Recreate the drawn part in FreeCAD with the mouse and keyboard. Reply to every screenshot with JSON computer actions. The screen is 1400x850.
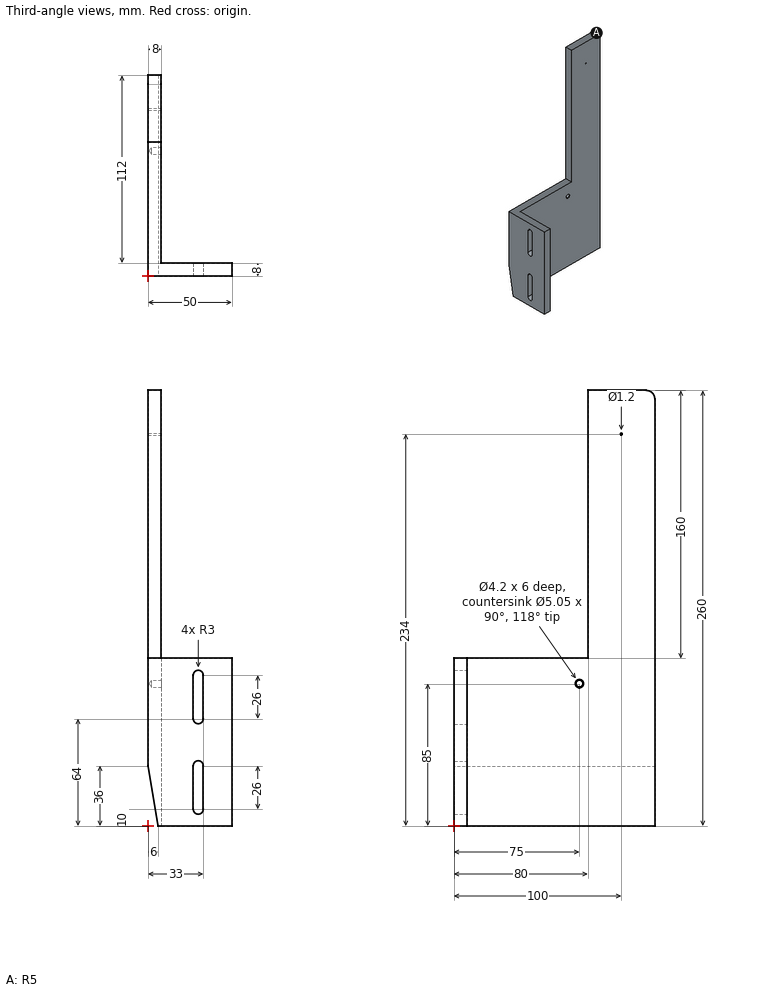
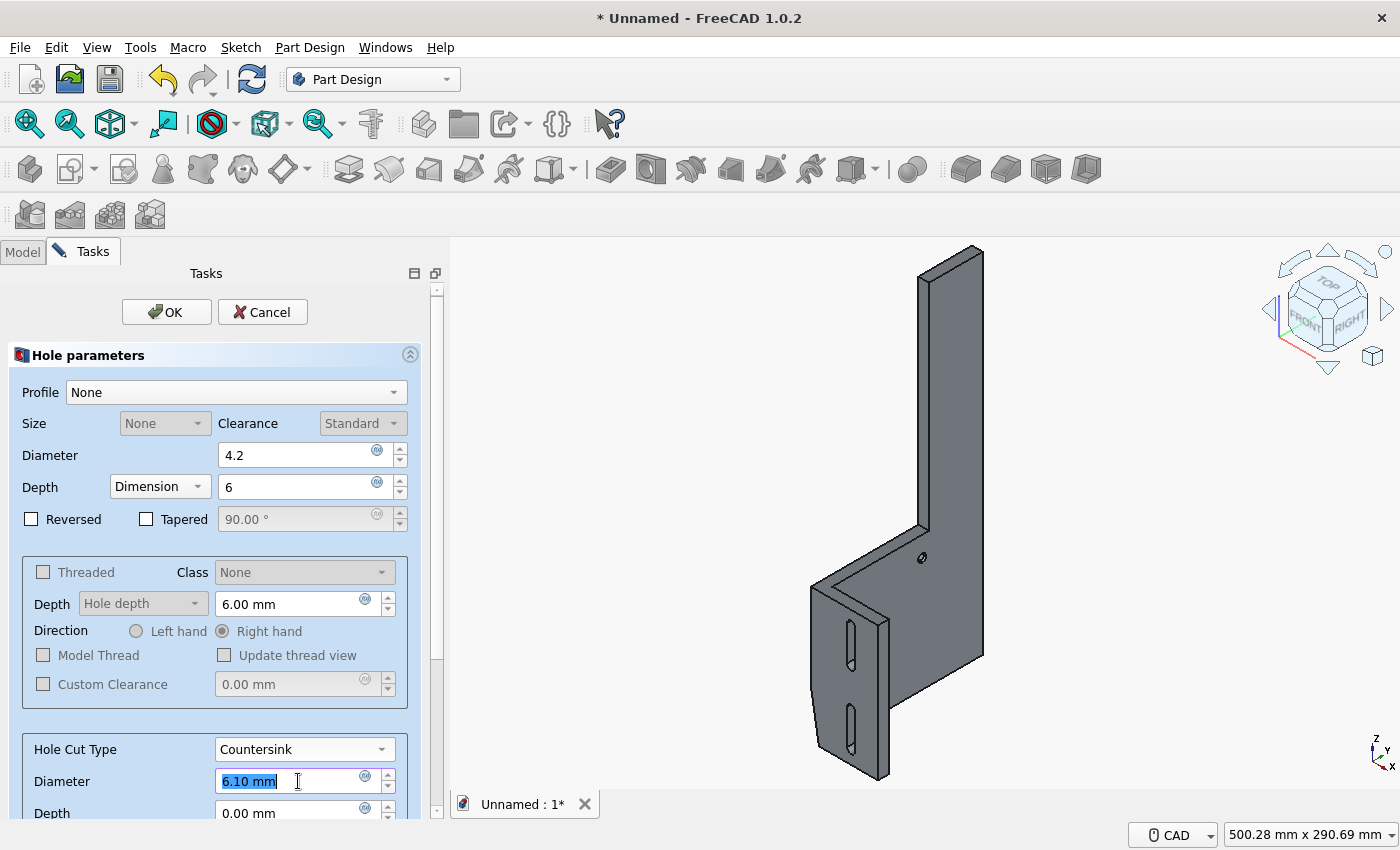
{"action": "type", "text": "5.05"}
{"action": "key", "text": "Tab"}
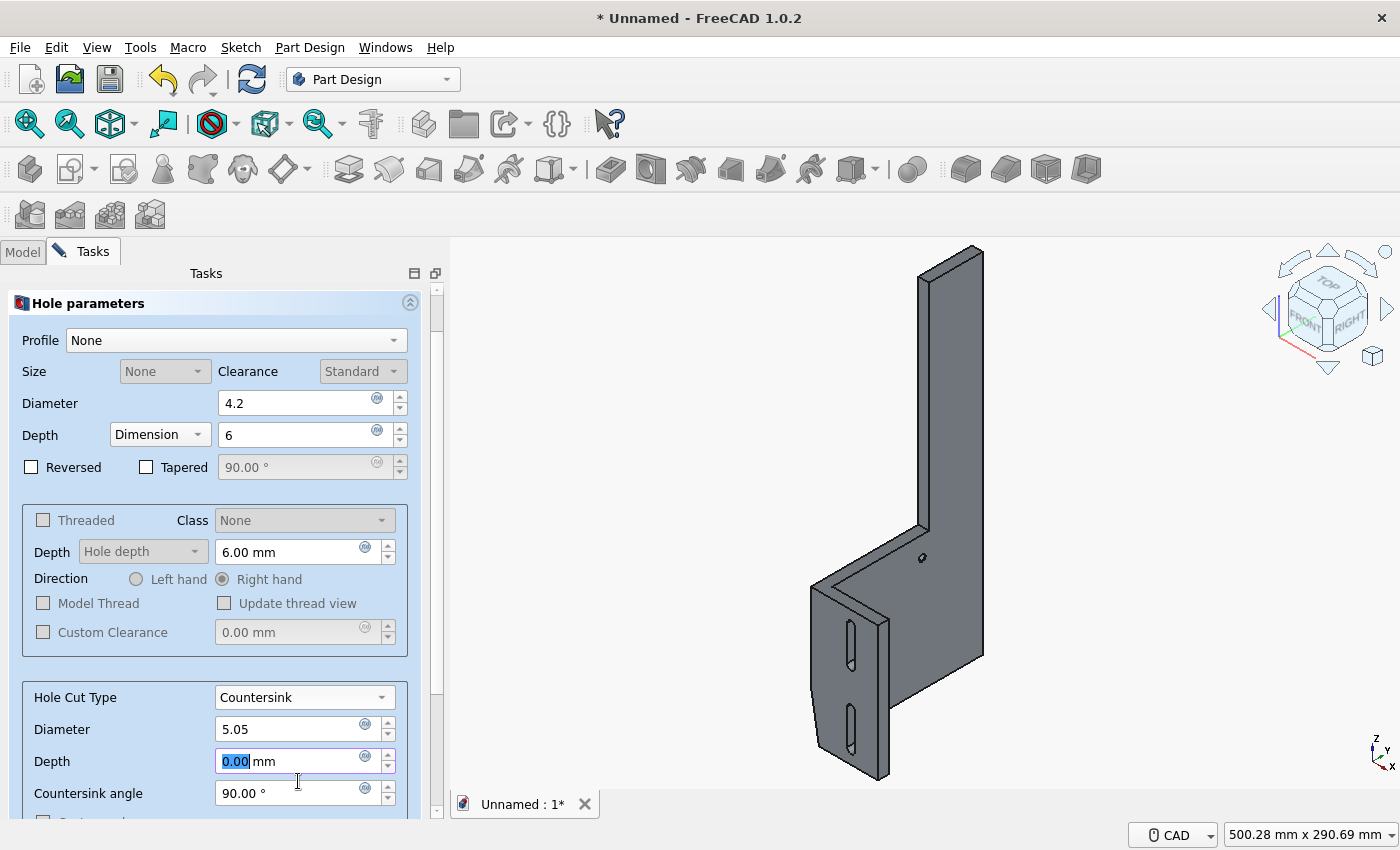
{"action": "scroll", "coordinate": [437, 550], "scroll_direction": "up", "scroll_amount": 2}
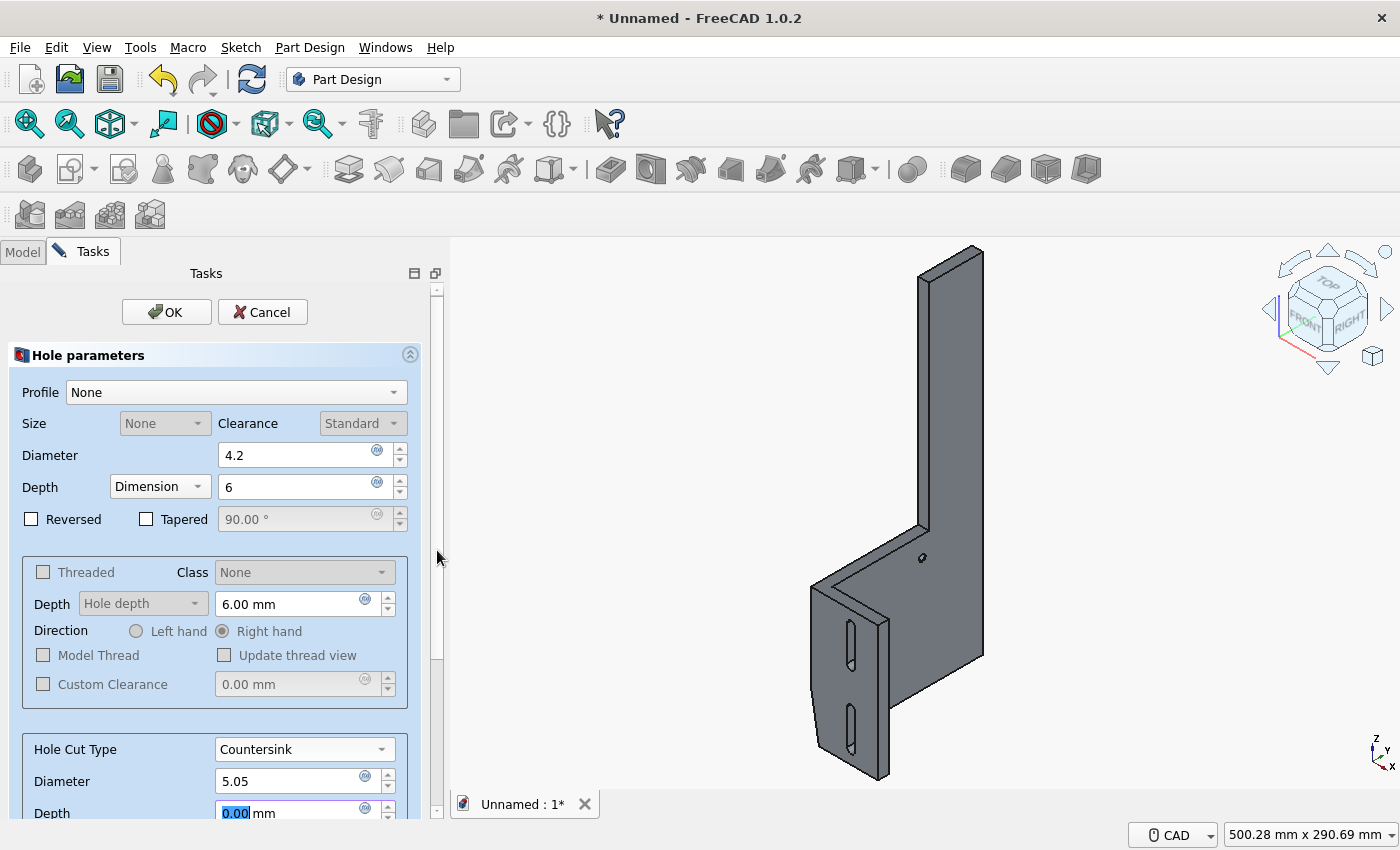
{"action": "left_click", "coordinate": [167, 312]}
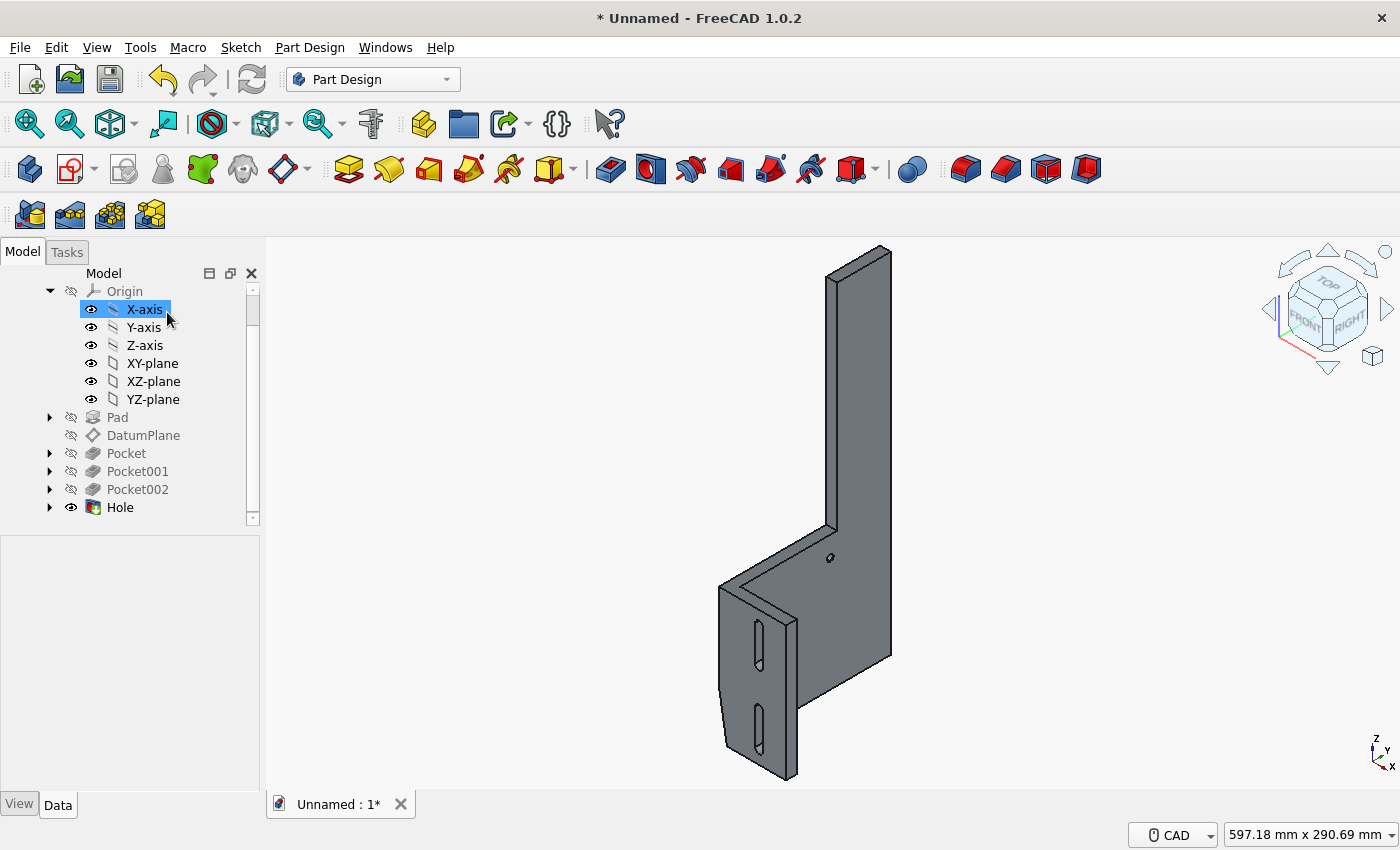
{"action": "key", "text": "2"}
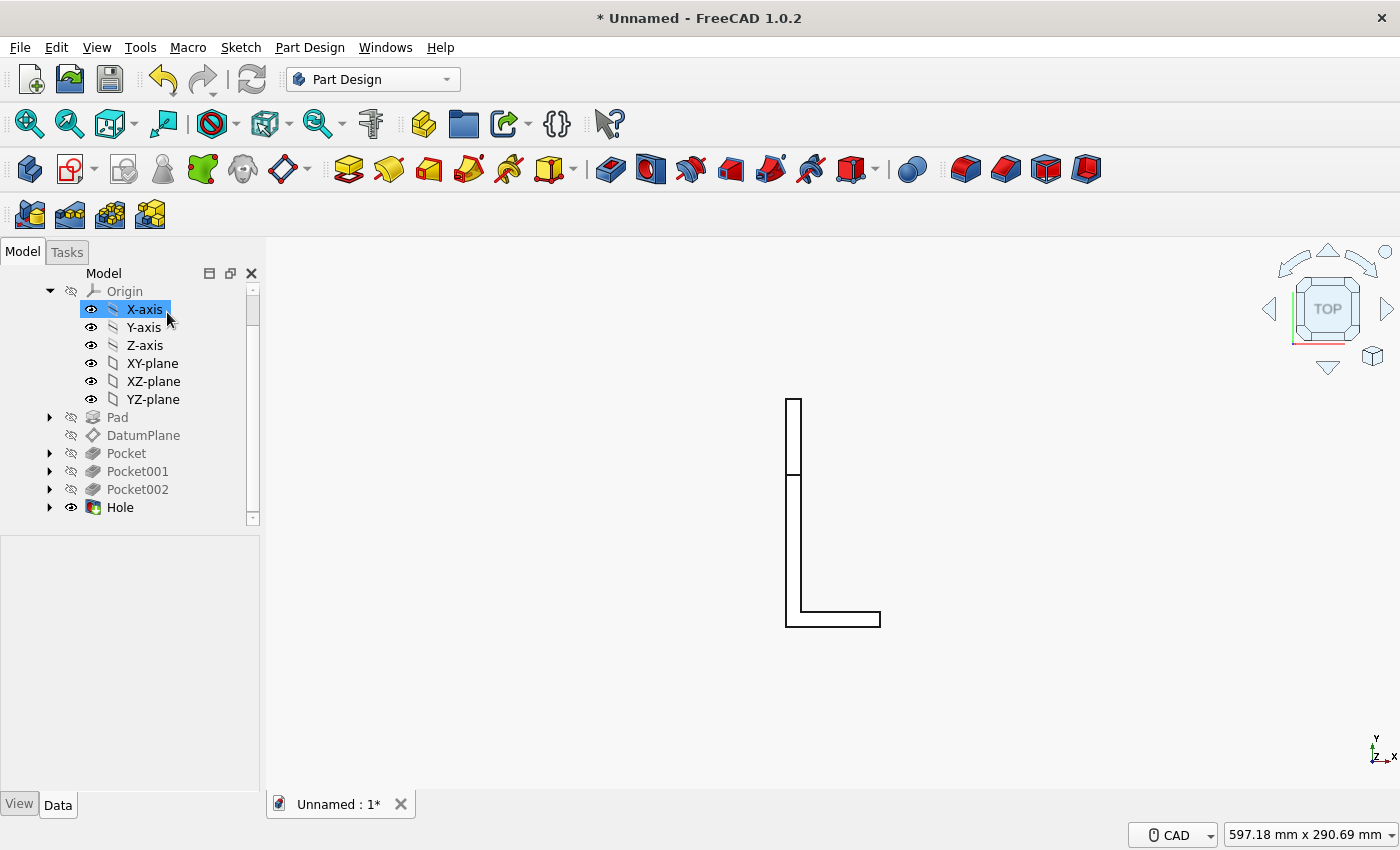
{"action": "left_click", "coordinate": [30, 124]}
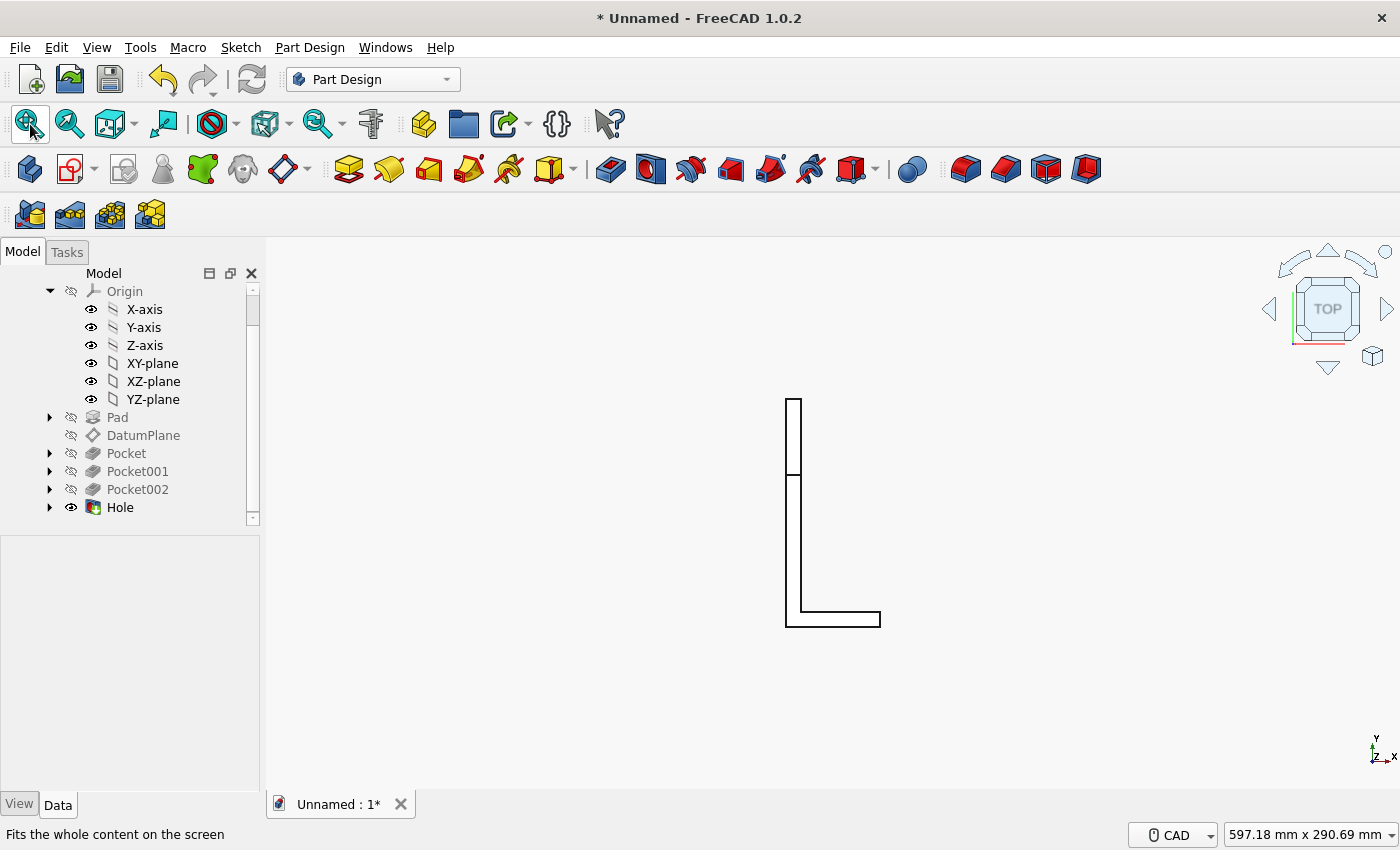
{"action": "left_click", "coordinate": [793, 398]}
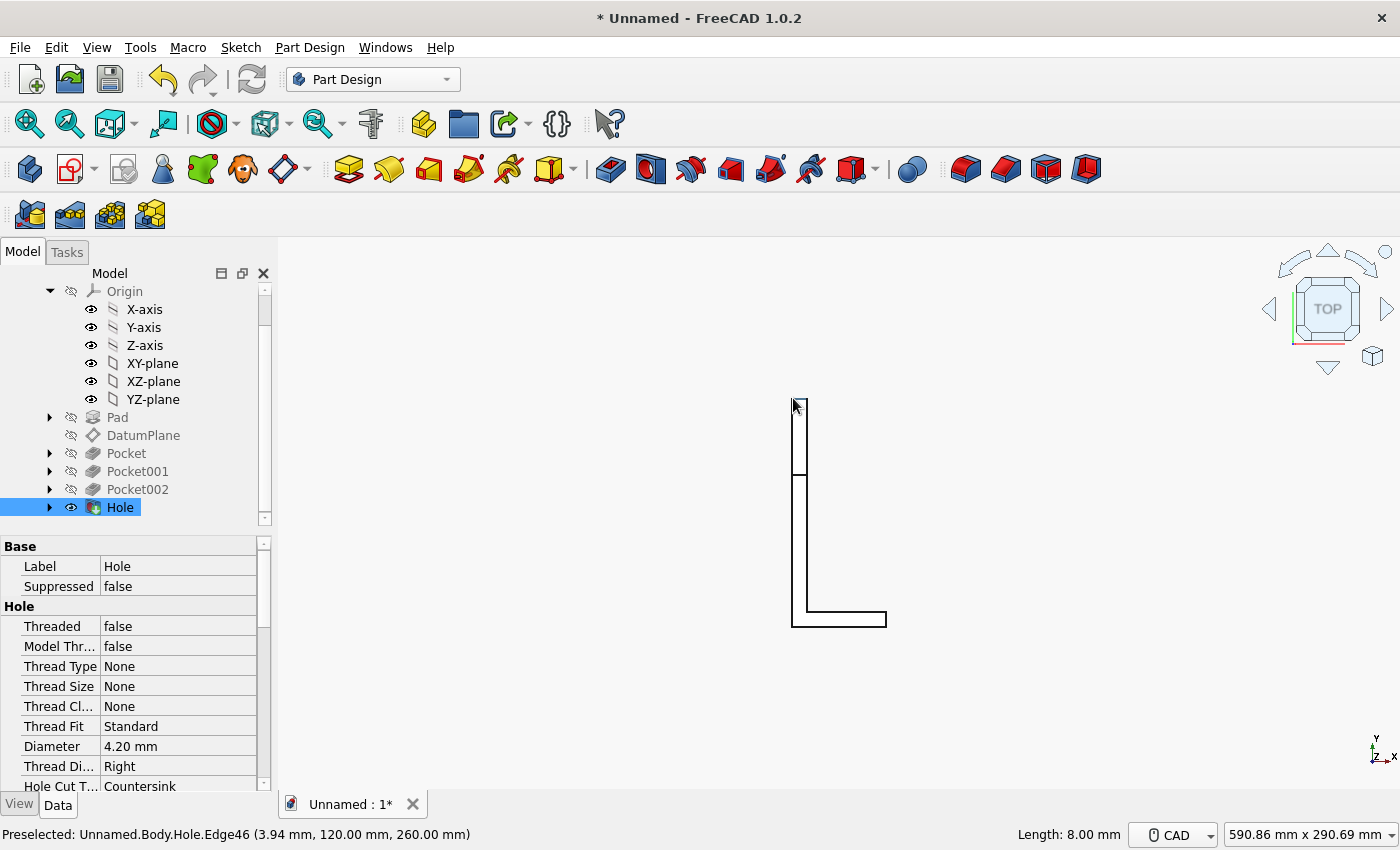
{"action": "left_click", "coordinate": [966, 170]}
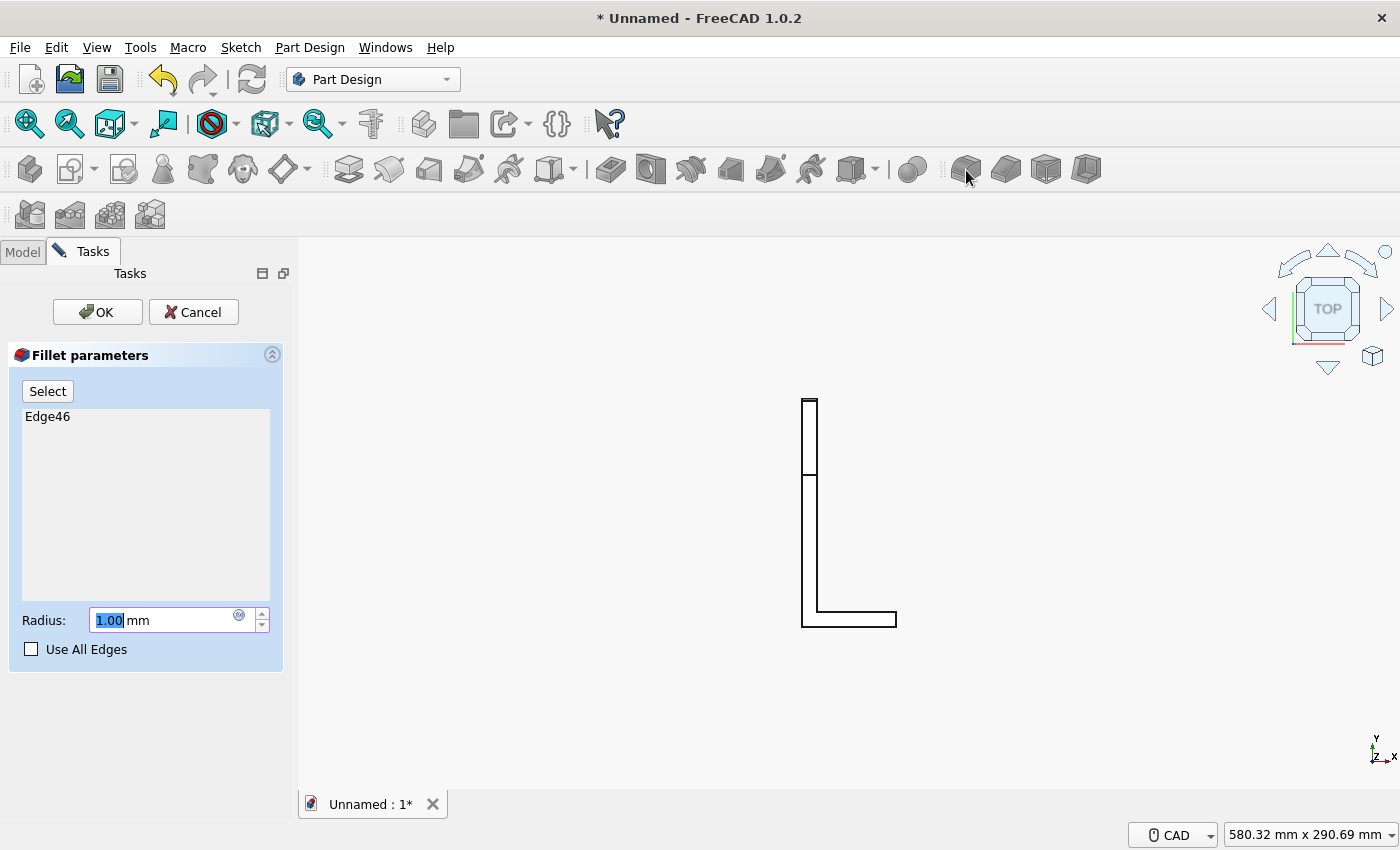
{"action": "type", "text": "5"}
{"action": "key", "text": "Tab"}